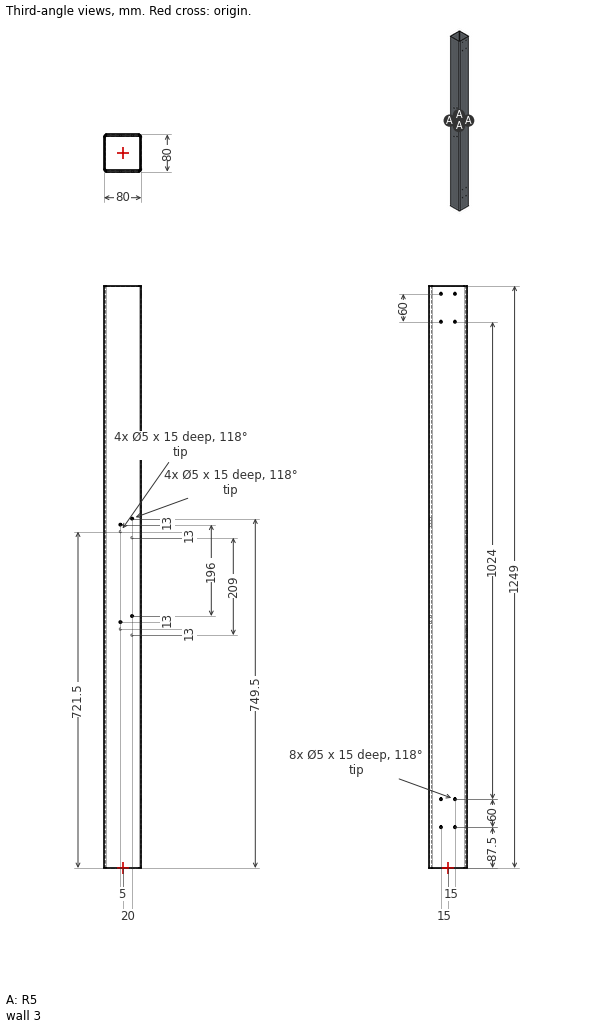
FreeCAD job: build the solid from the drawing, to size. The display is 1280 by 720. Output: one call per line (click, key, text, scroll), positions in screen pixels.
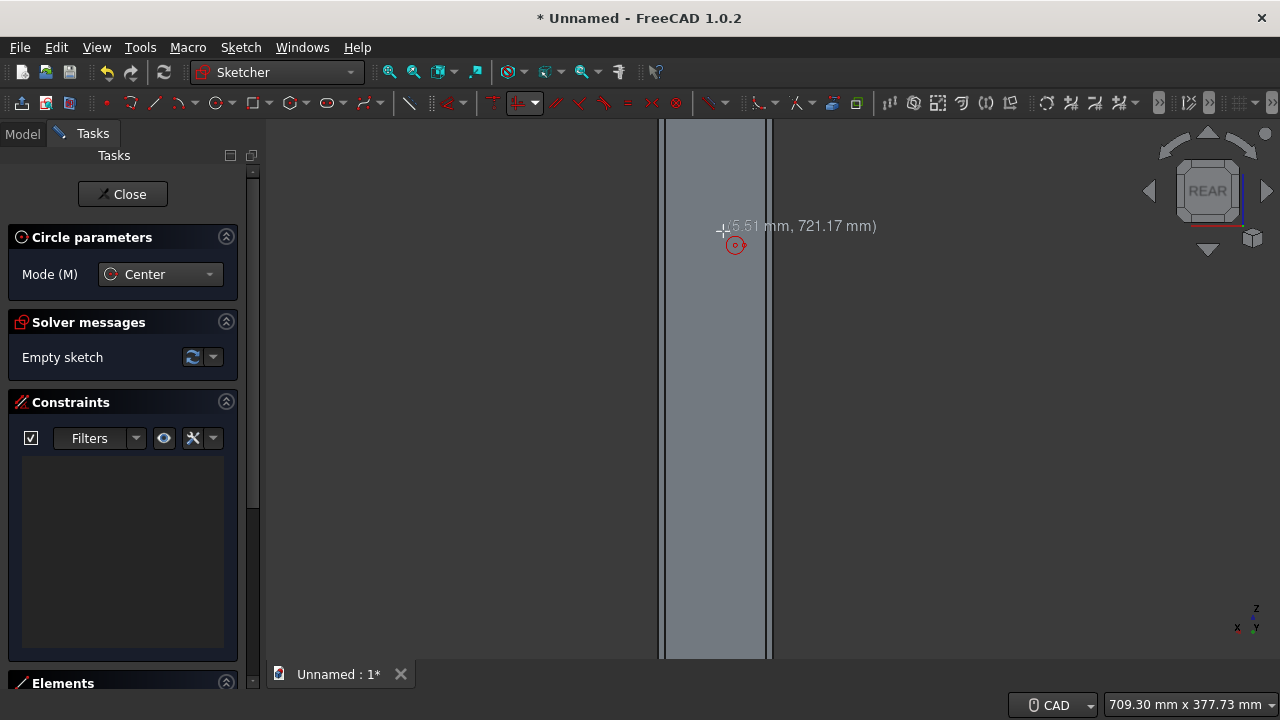
scroll(723, 231, up, 4)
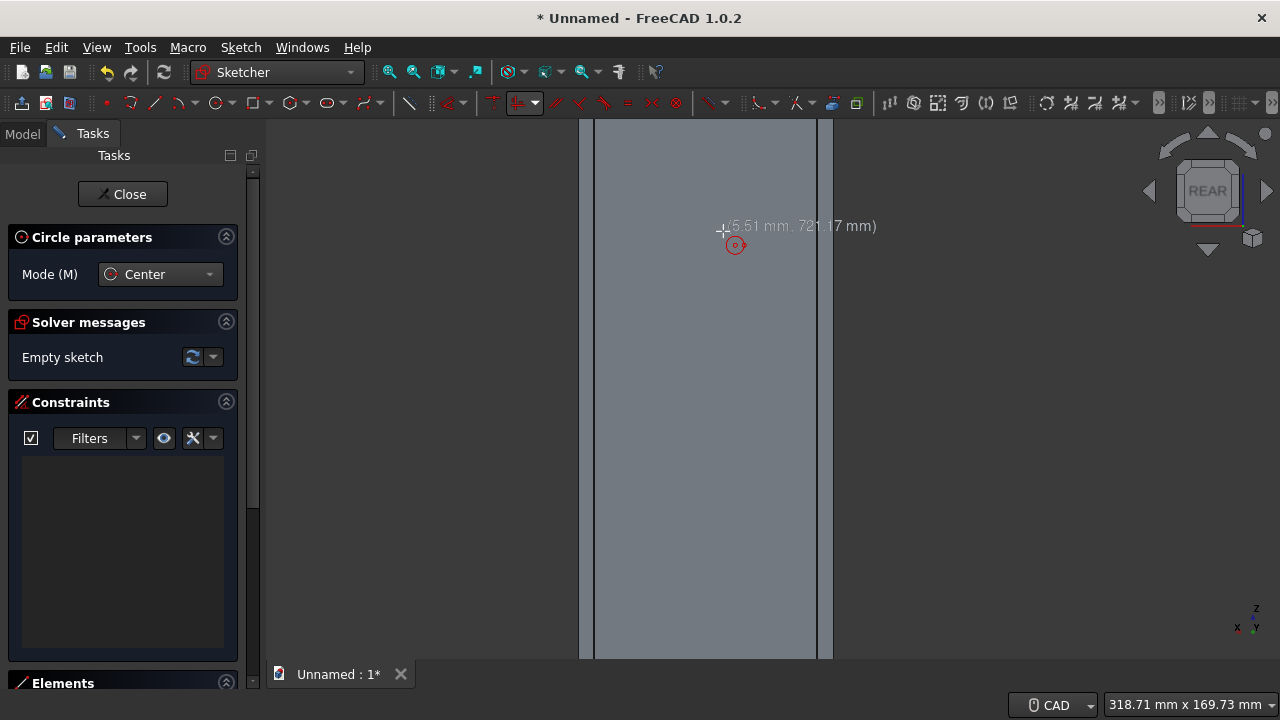
click(722, 230)
move(727, 225)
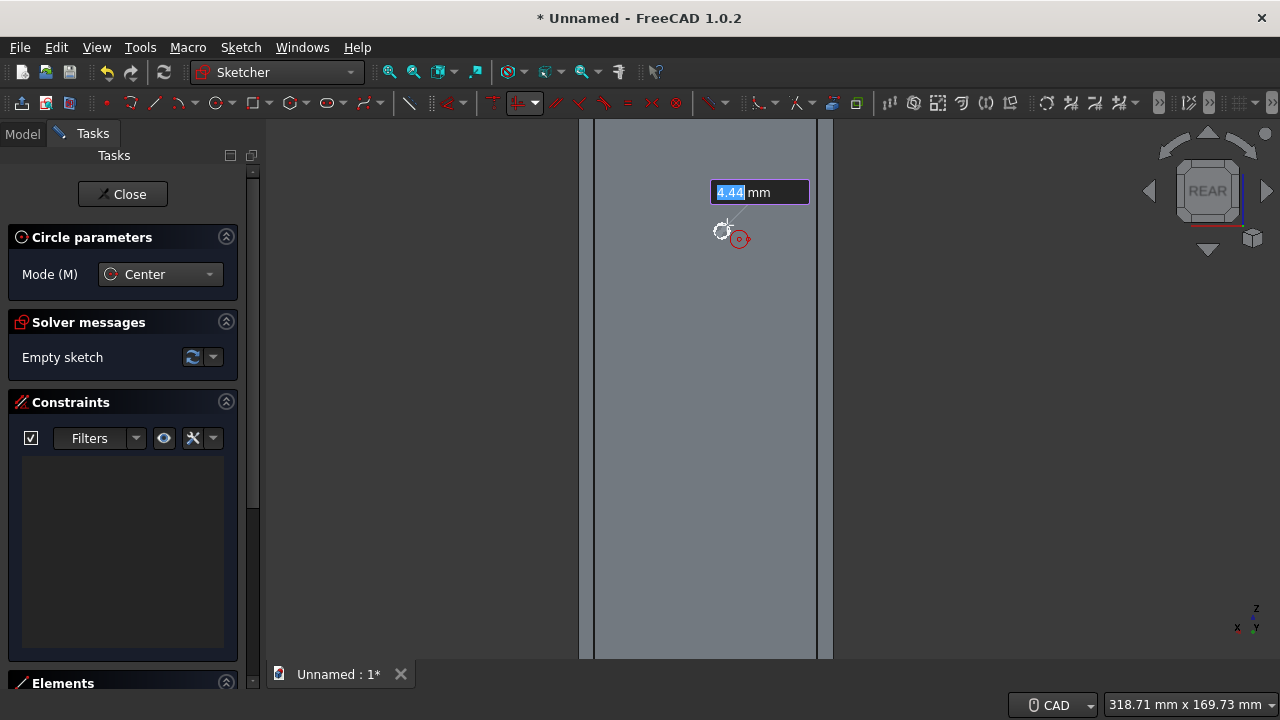
text(5)
key(Return)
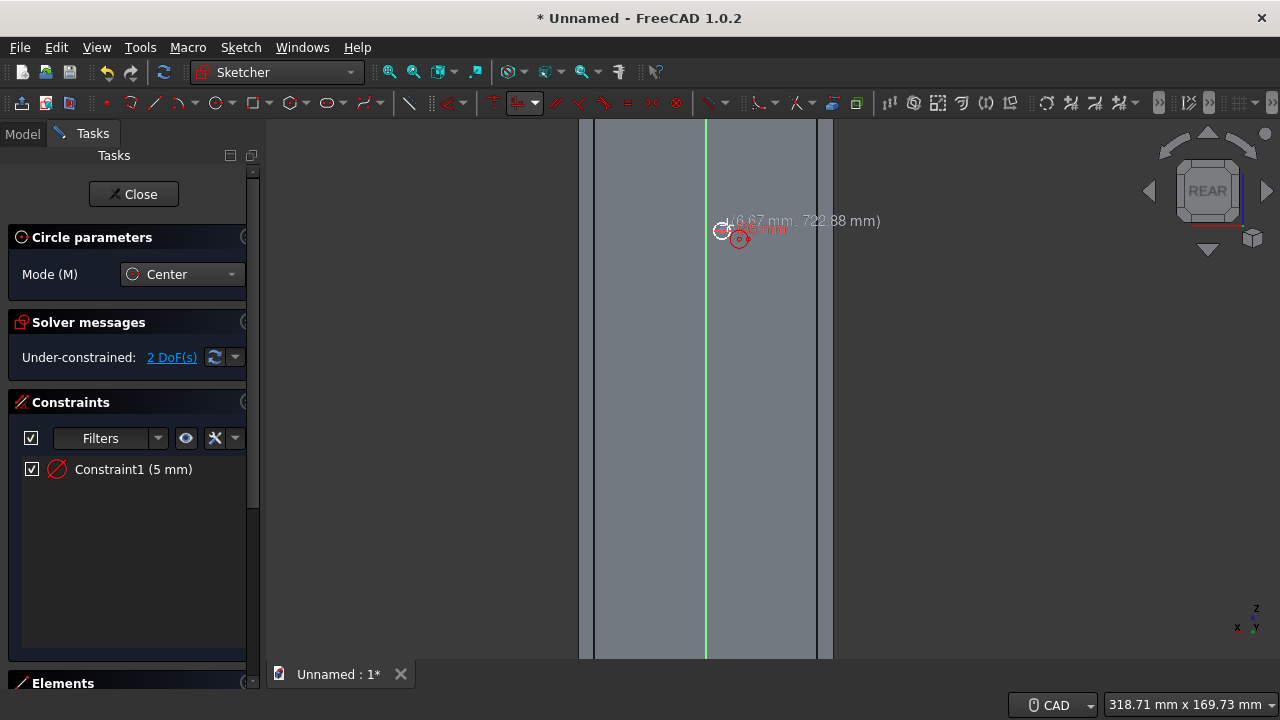
scroll(642, 272, up, 6)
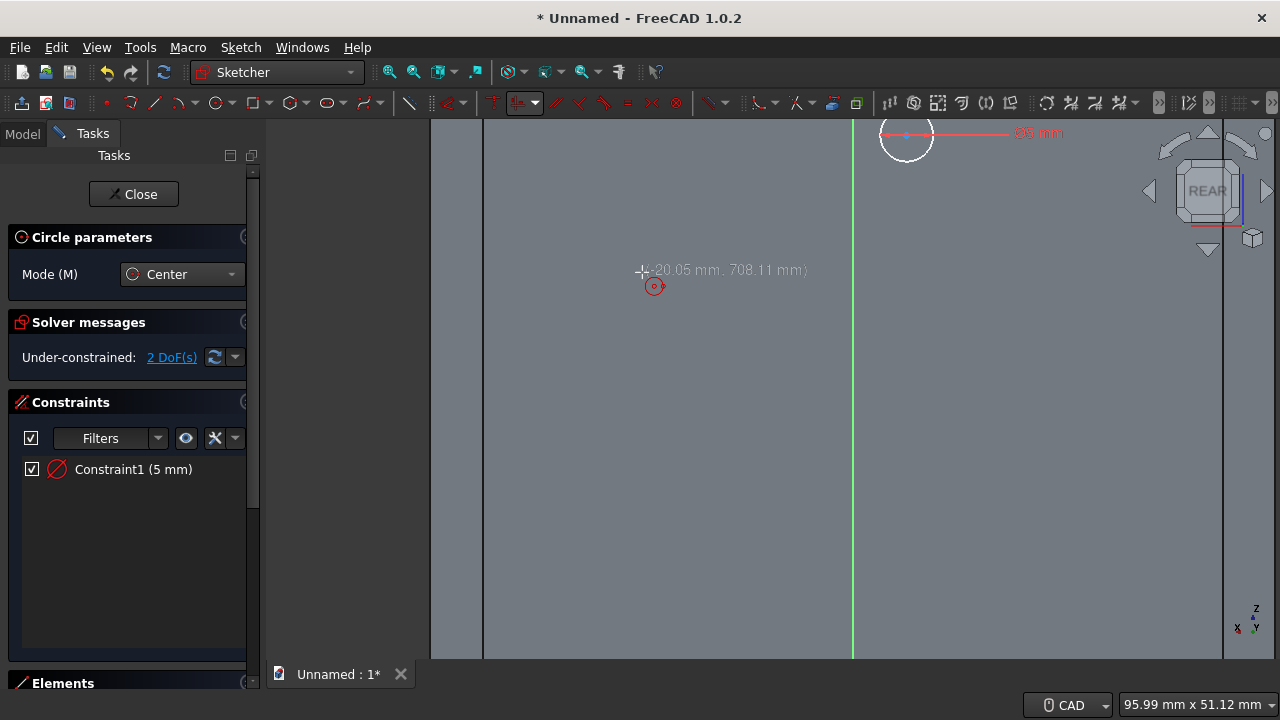
scroll(694, 246, down, 10)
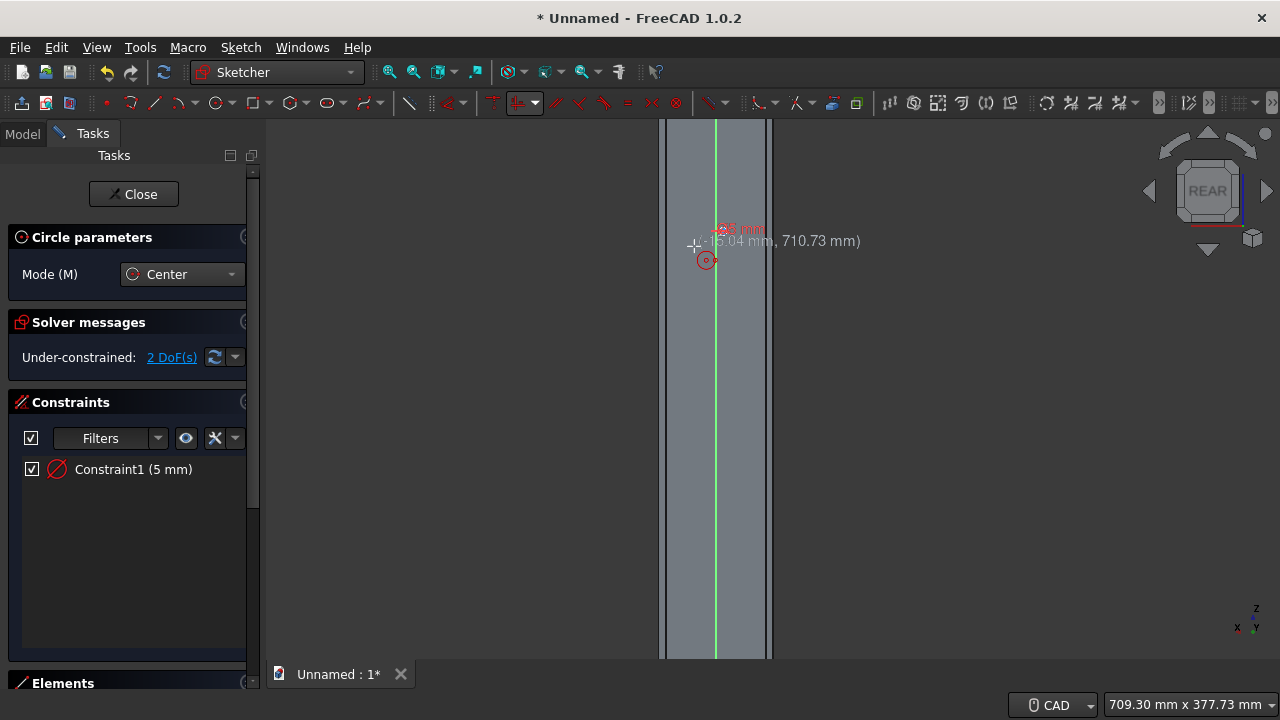
click(687, 250)
move(690, 247)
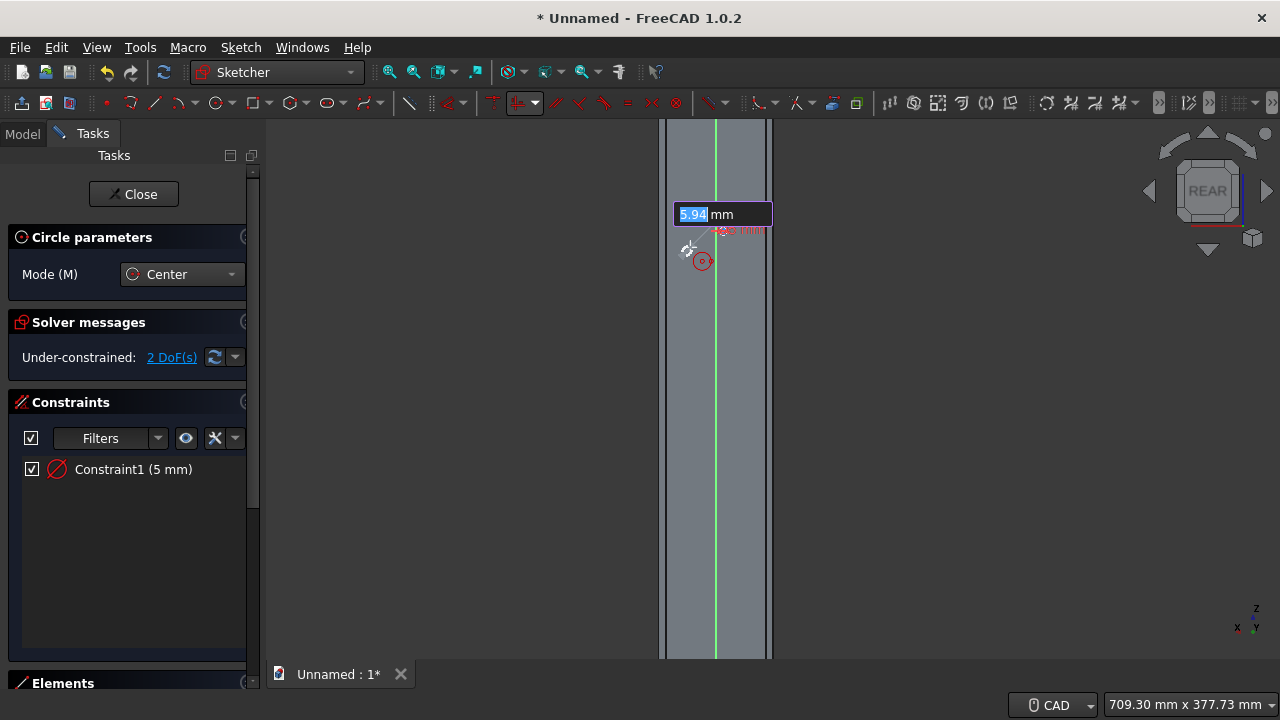
text(5)
key(Return)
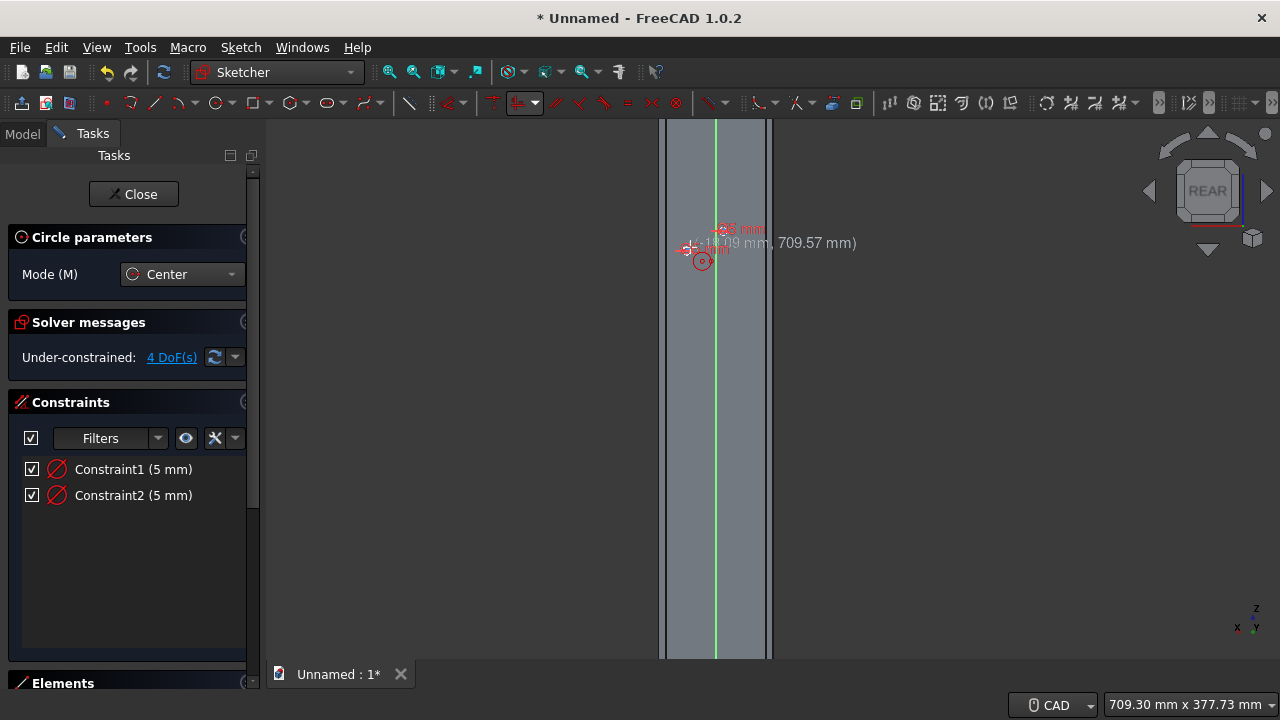
scroll(687, 548, up, 10)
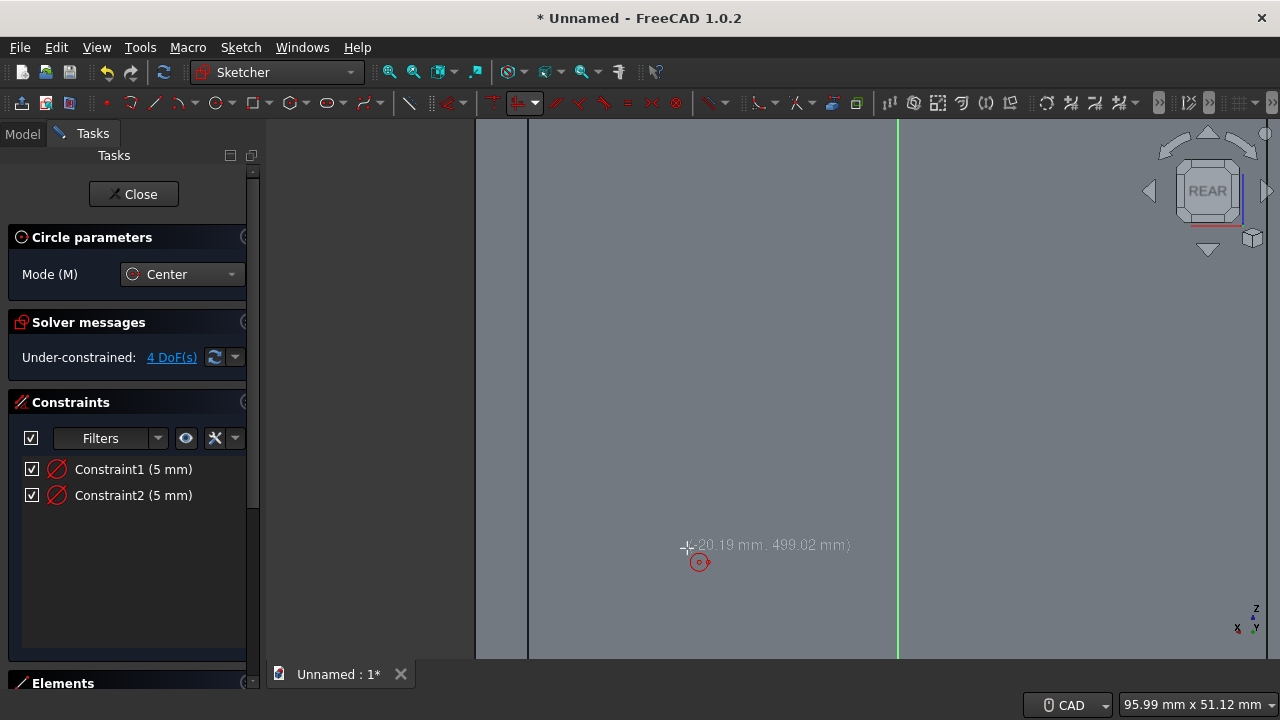
scroll(687, 548, down, 10)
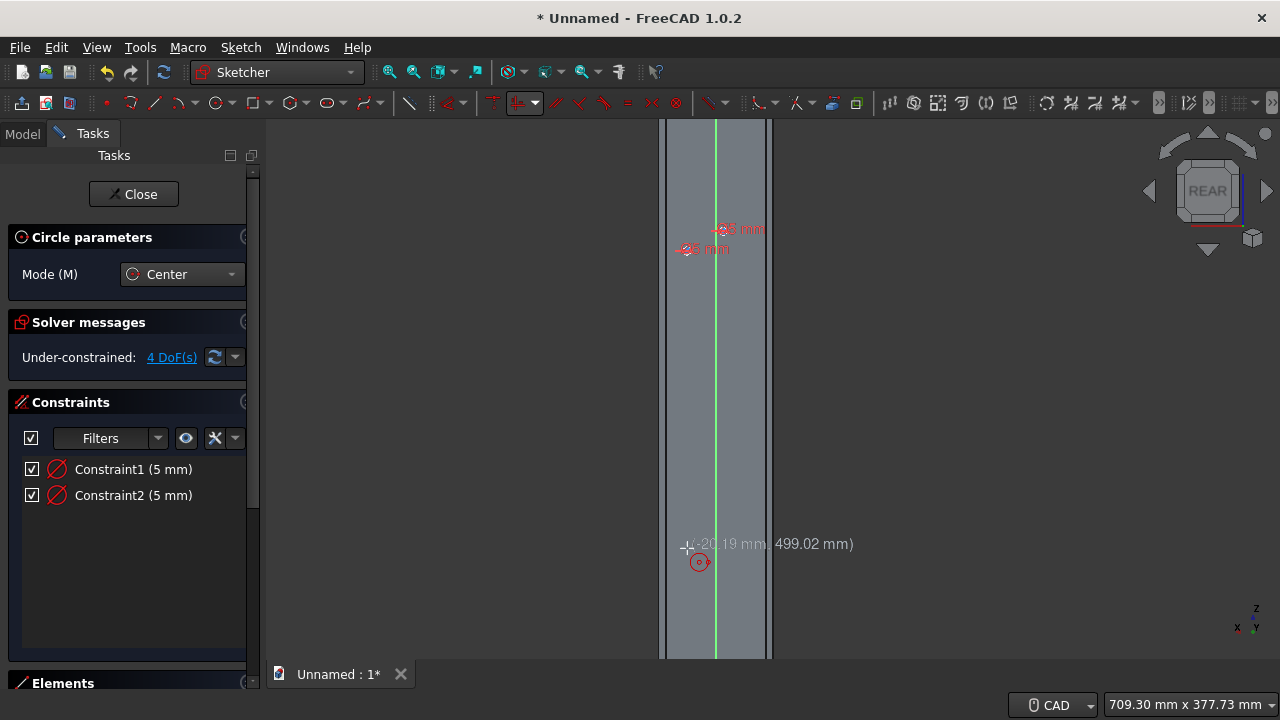
click(687, 548)
move(690, 546)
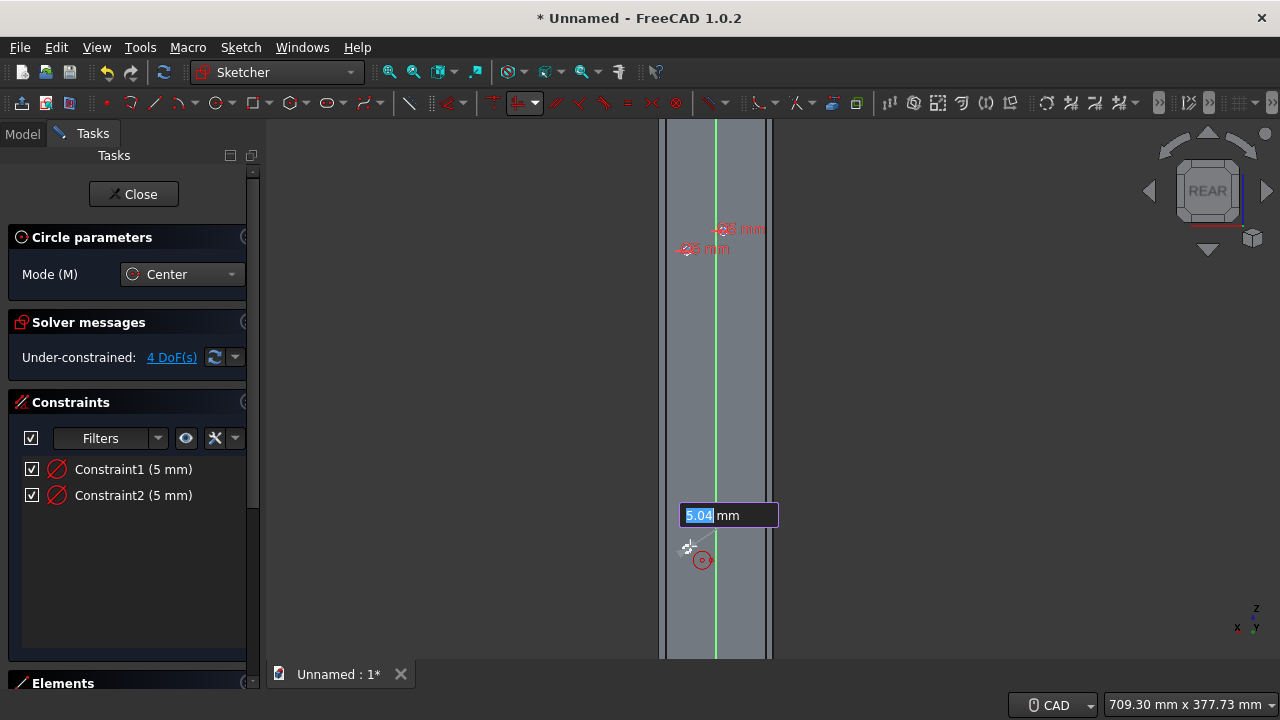
text(5)
key(Return)